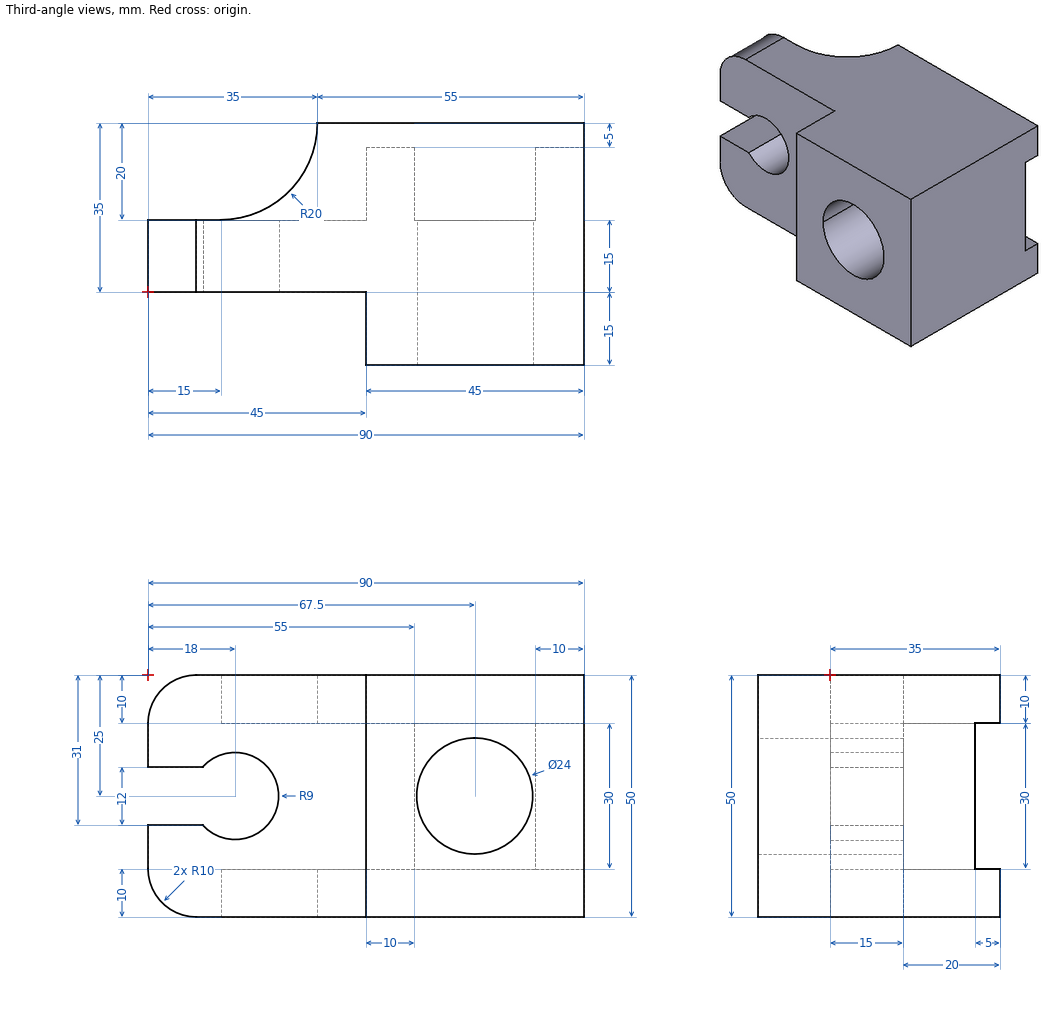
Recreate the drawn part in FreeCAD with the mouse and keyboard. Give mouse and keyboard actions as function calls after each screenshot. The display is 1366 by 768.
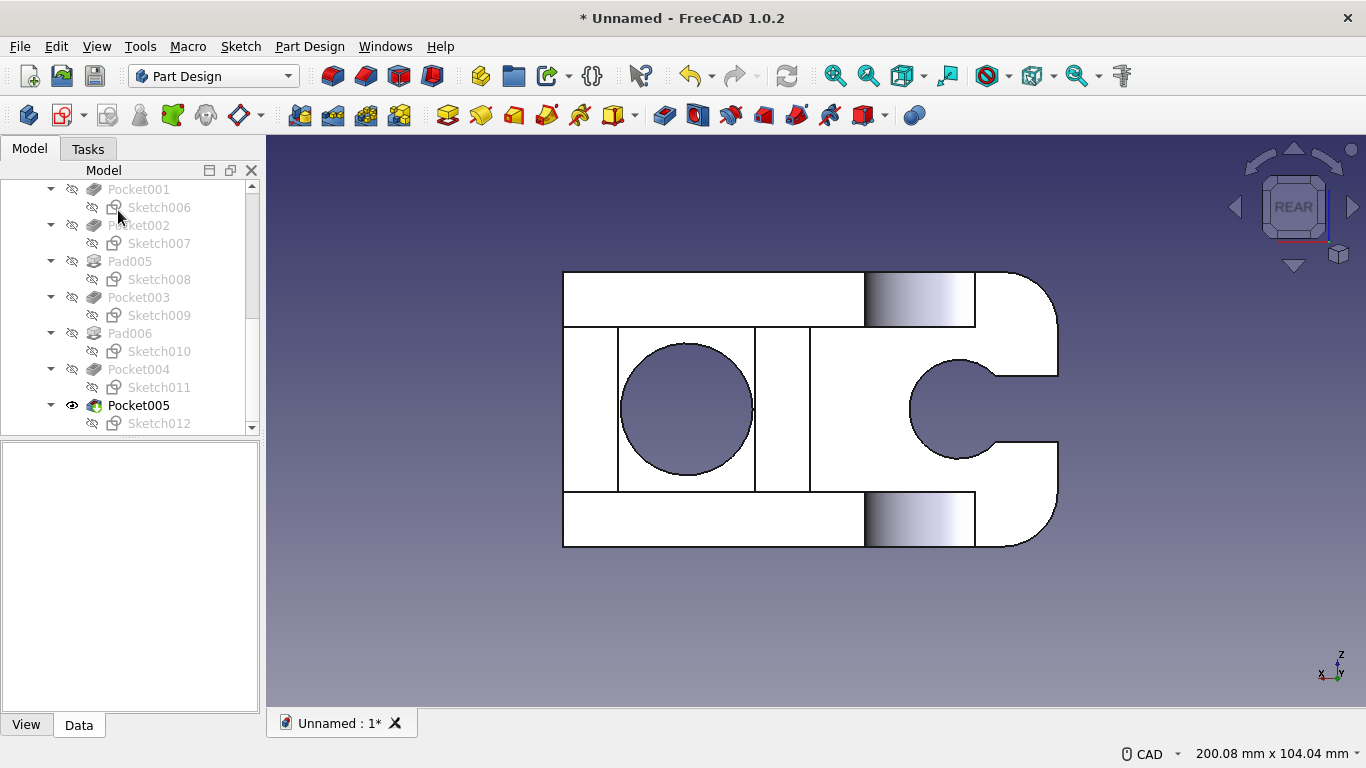
key(0)